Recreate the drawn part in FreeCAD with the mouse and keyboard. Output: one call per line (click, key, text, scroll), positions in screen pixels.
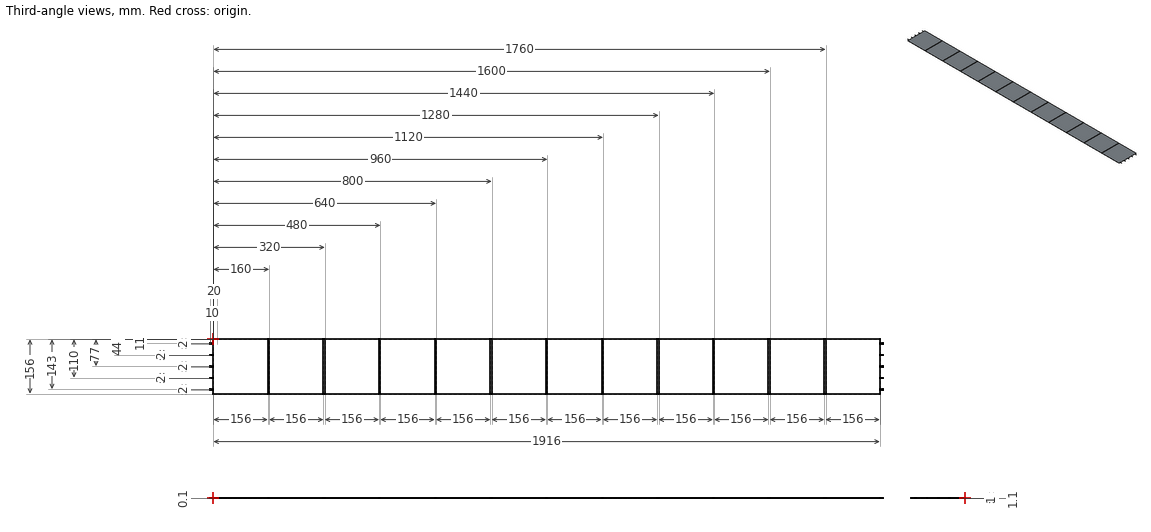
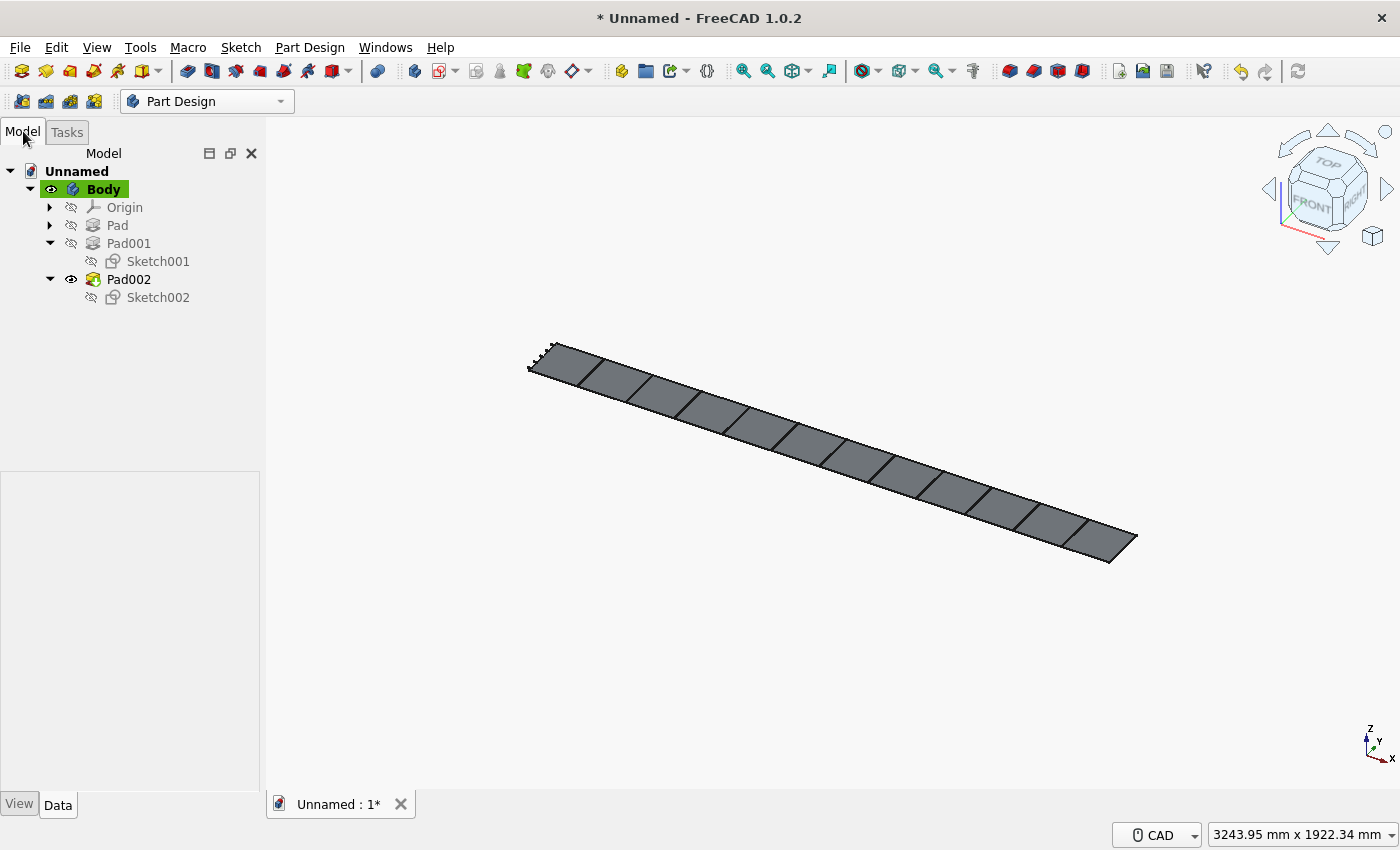
click(50, 207)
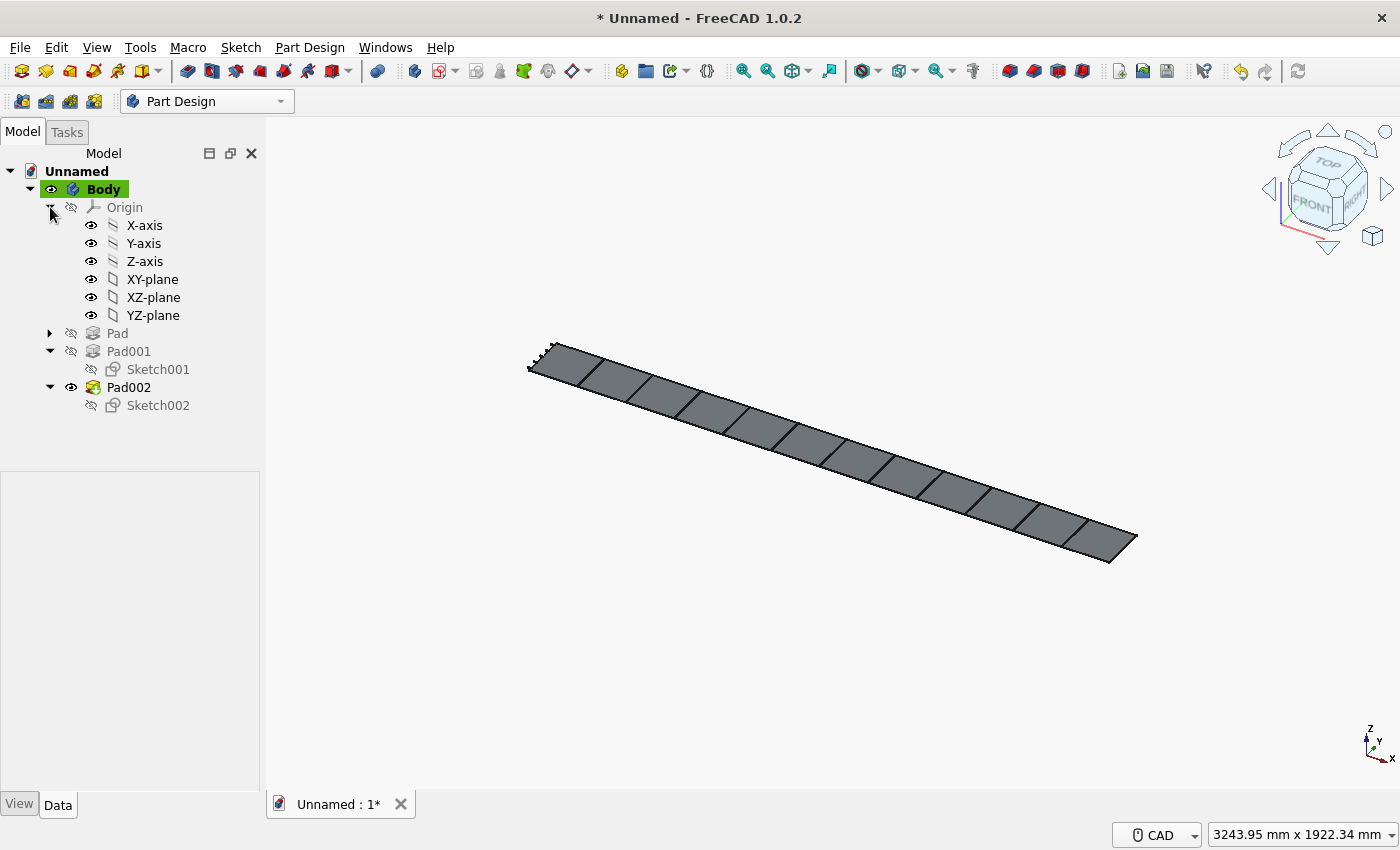
click(136, 315)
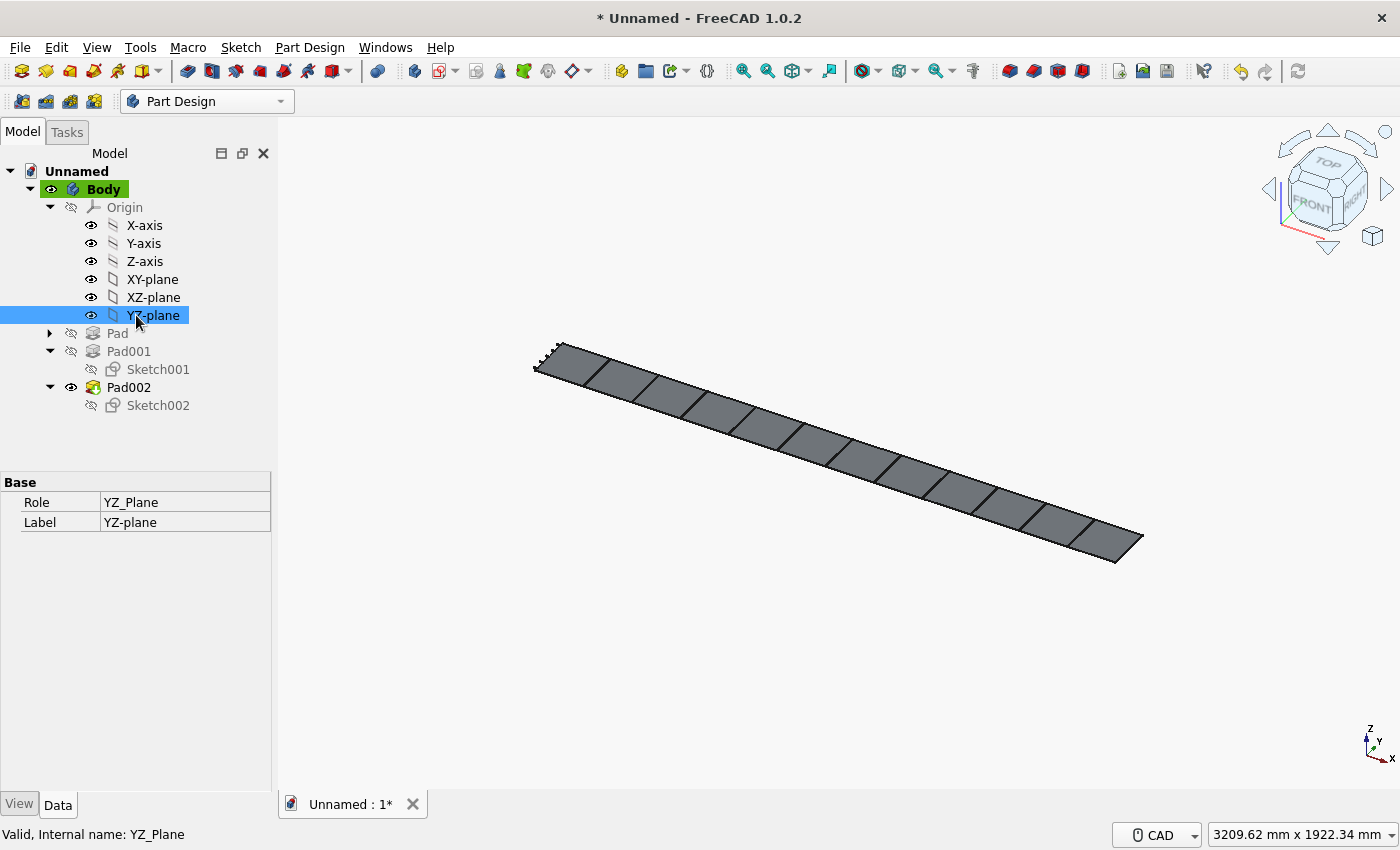
click(572, 72)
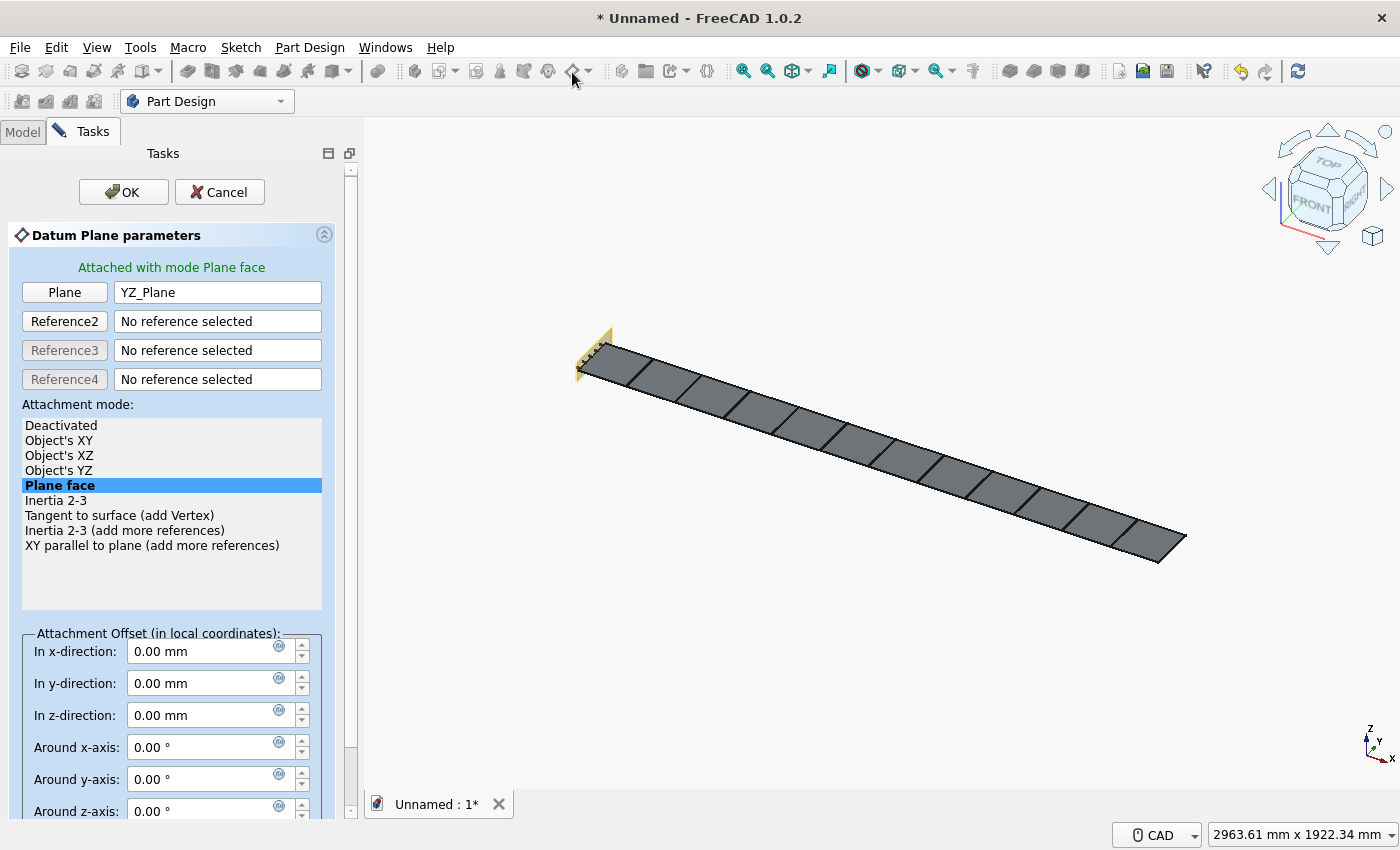
triple_click(210, 715)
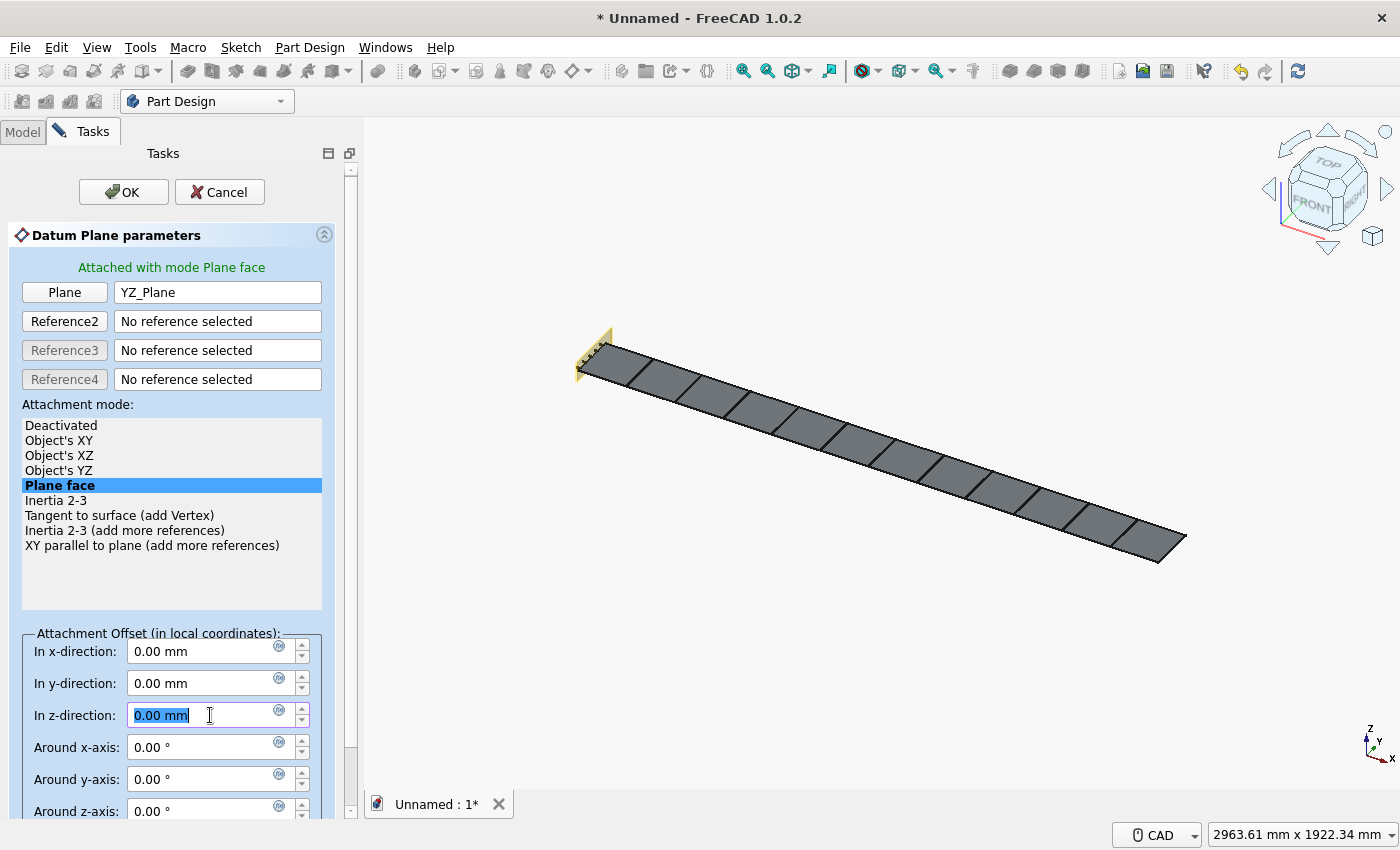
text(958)
key(Tab)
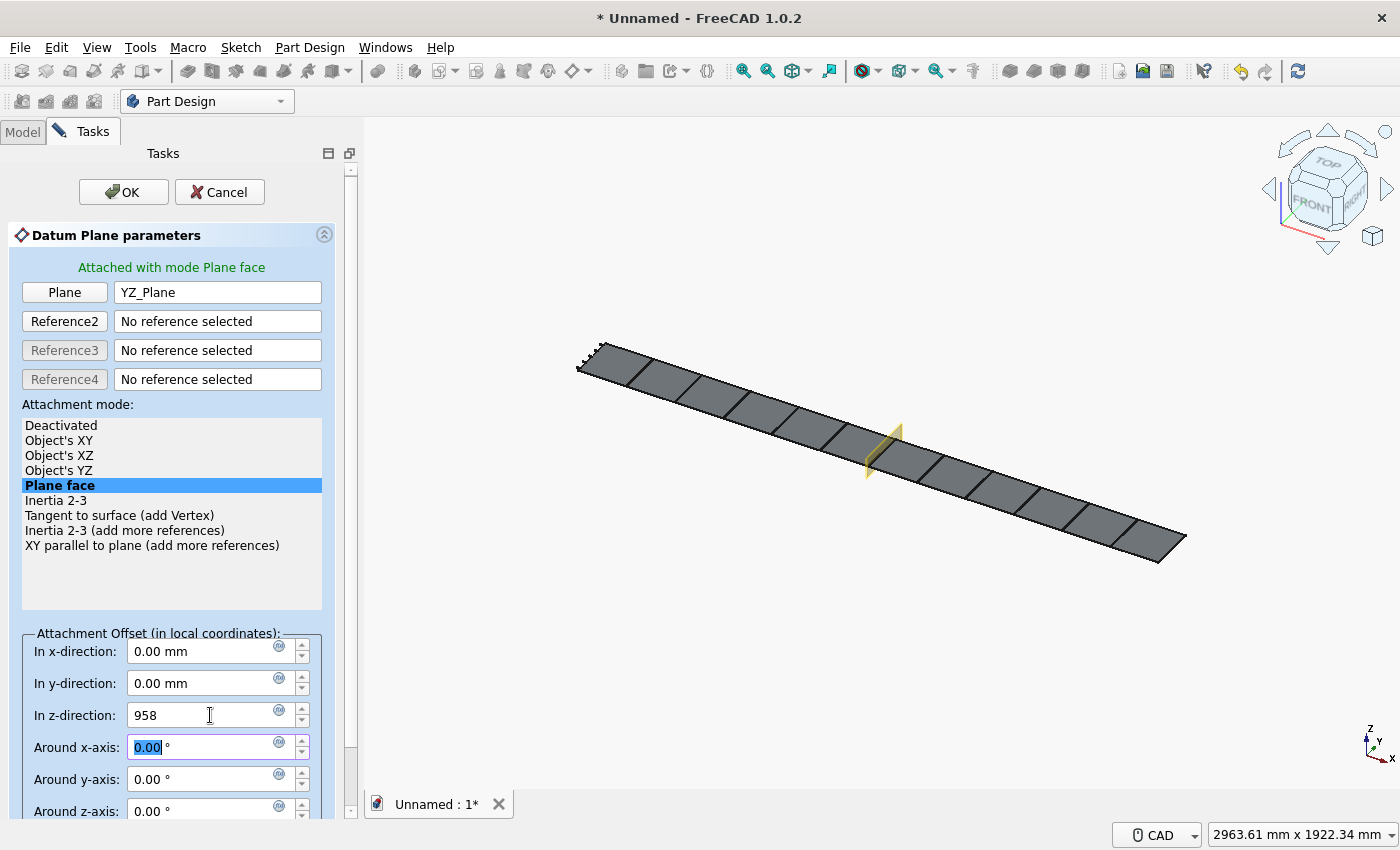
click(124, 192)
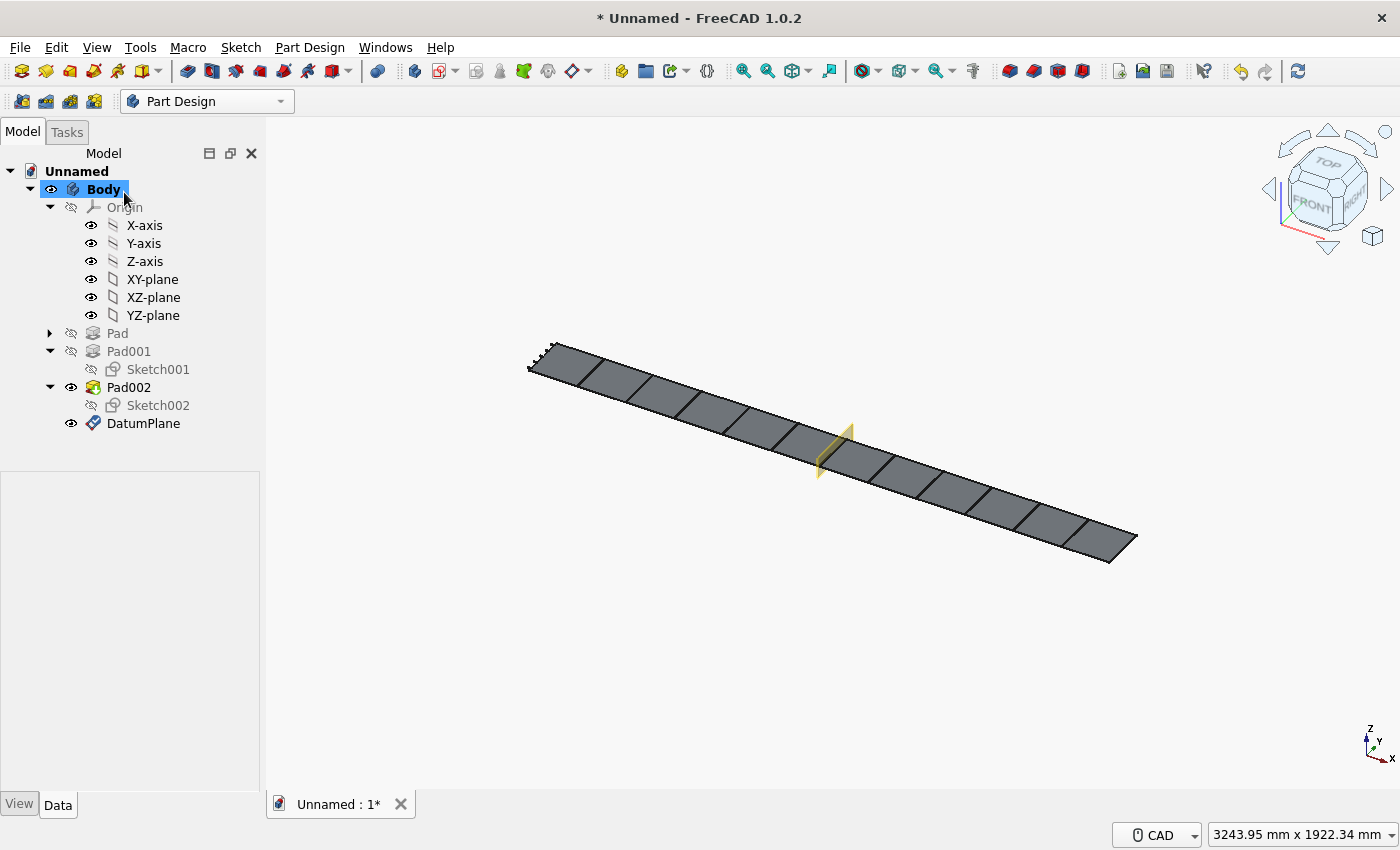
click(116, 387)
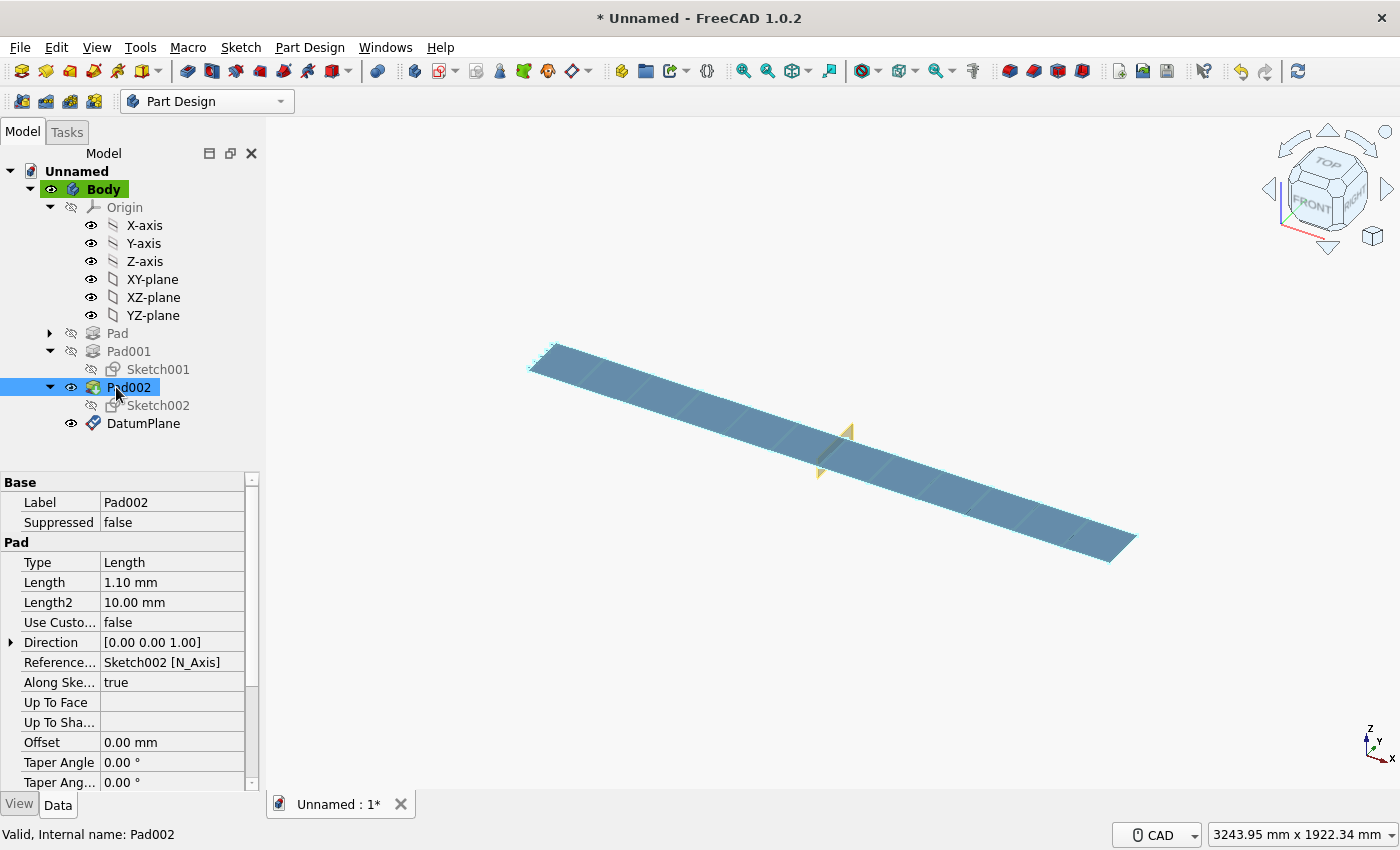
click(22, 102)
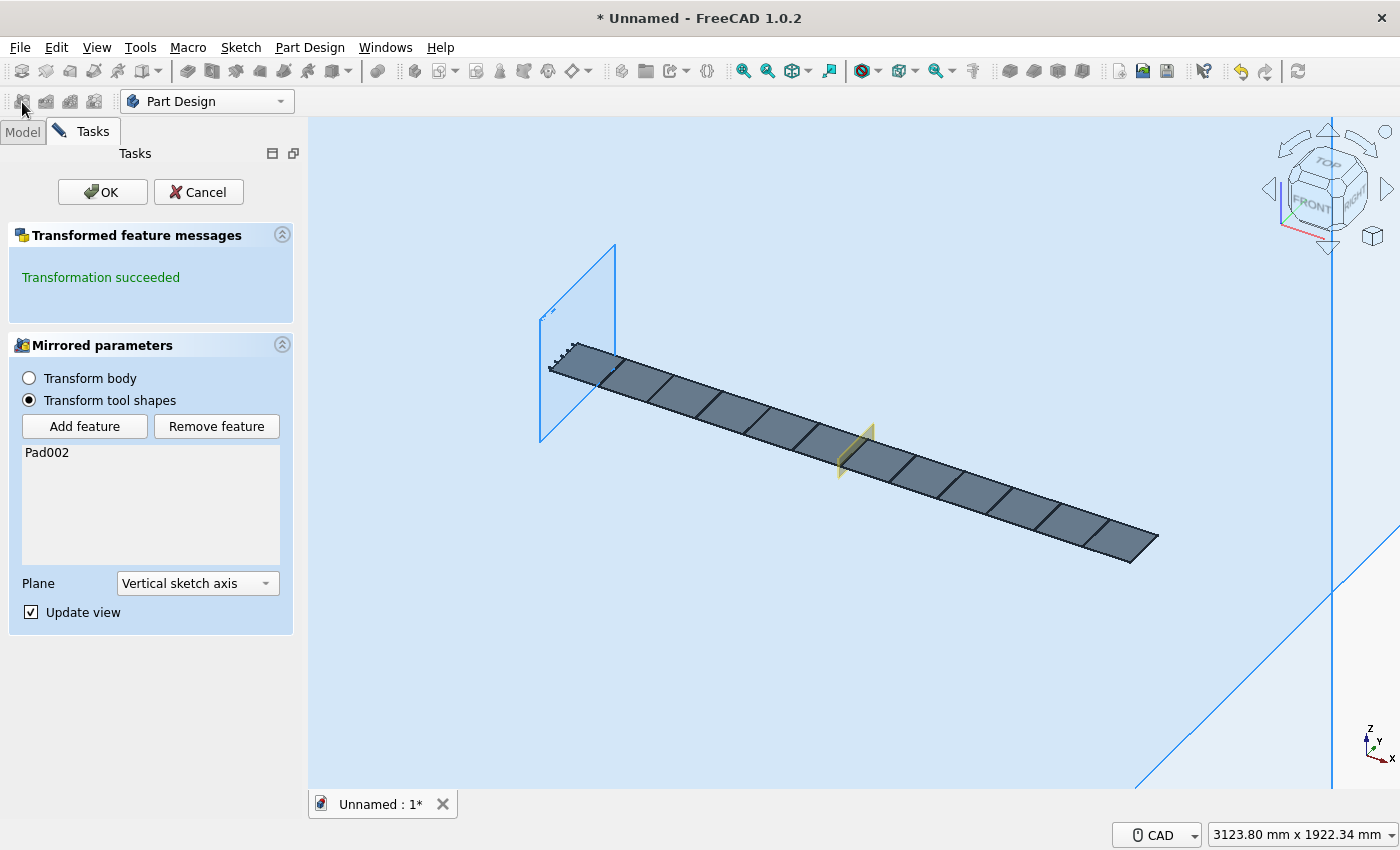
click(198, 584)